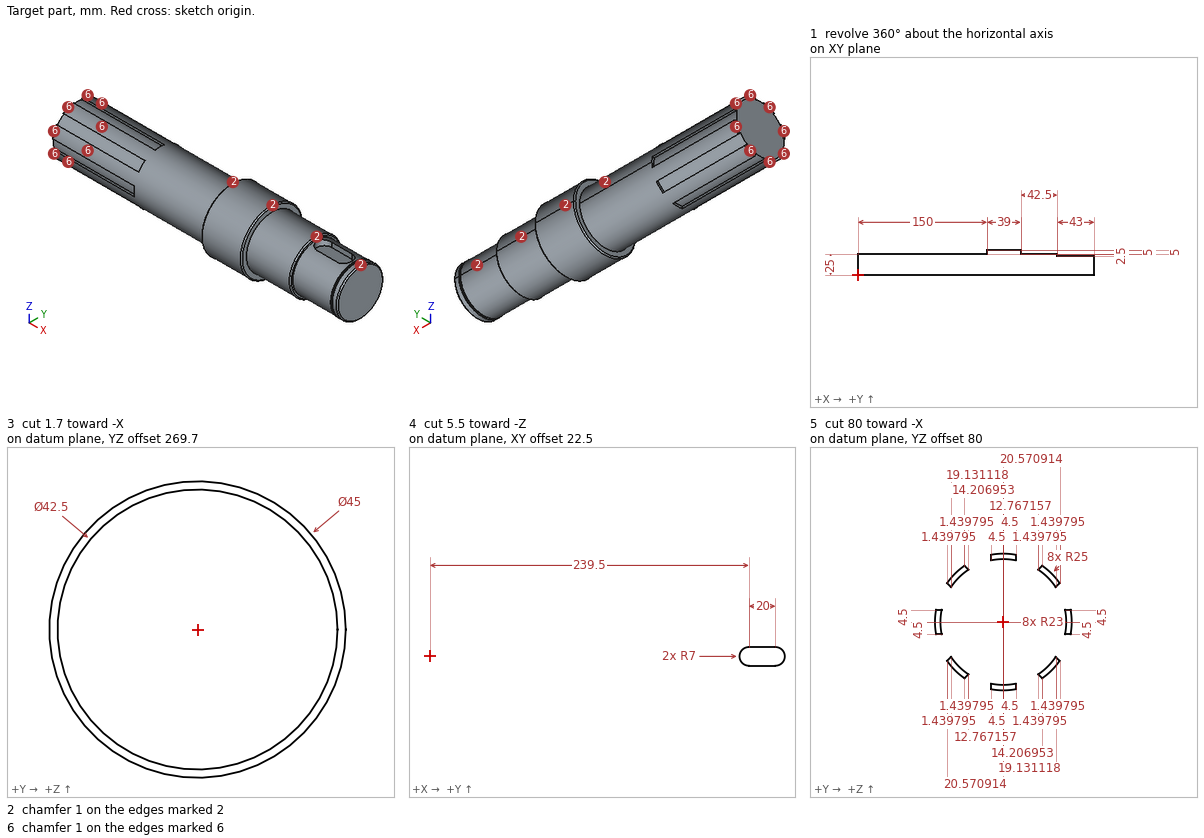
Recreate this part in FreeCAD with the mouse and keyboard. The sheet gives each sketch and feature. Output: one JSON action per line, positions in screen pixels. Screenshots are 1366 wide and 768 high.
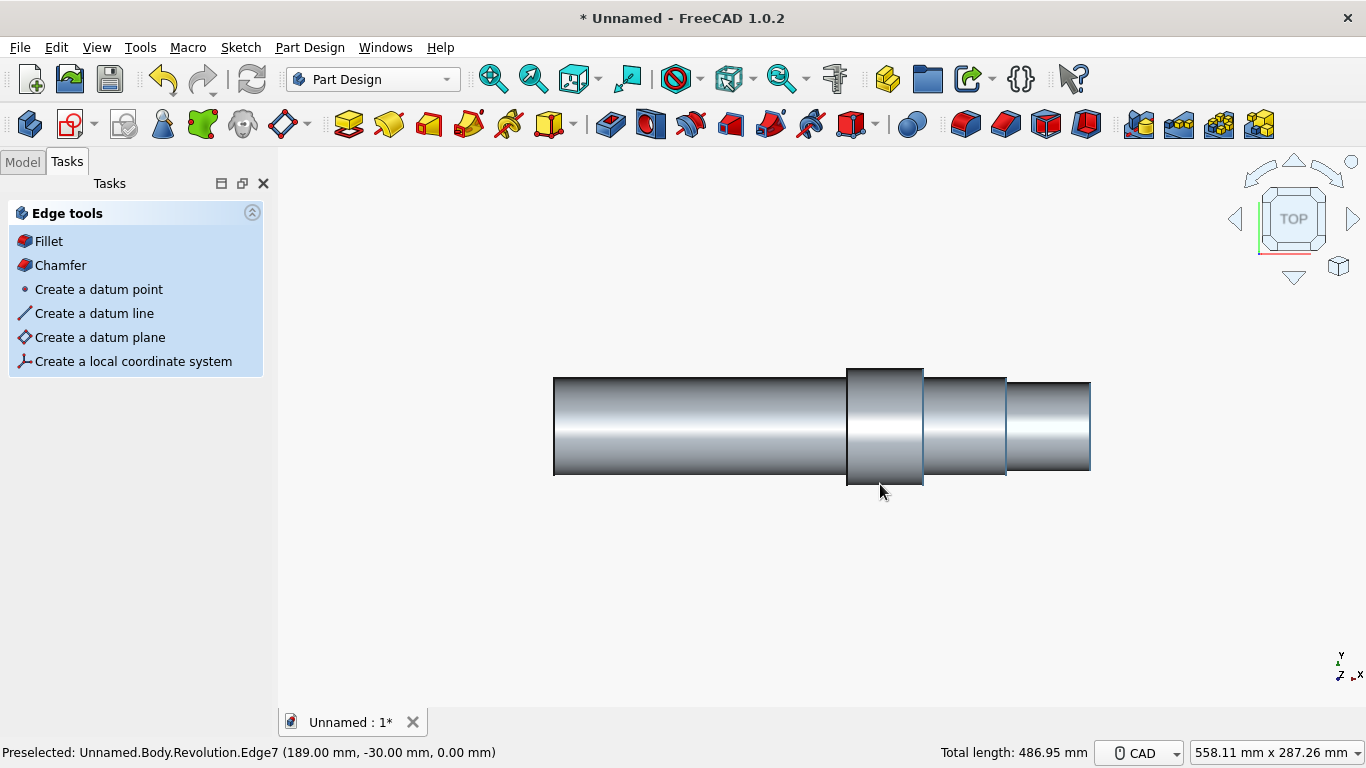
{"action": "left_click", "coordinate": [847, 473], "text": "ctrl"}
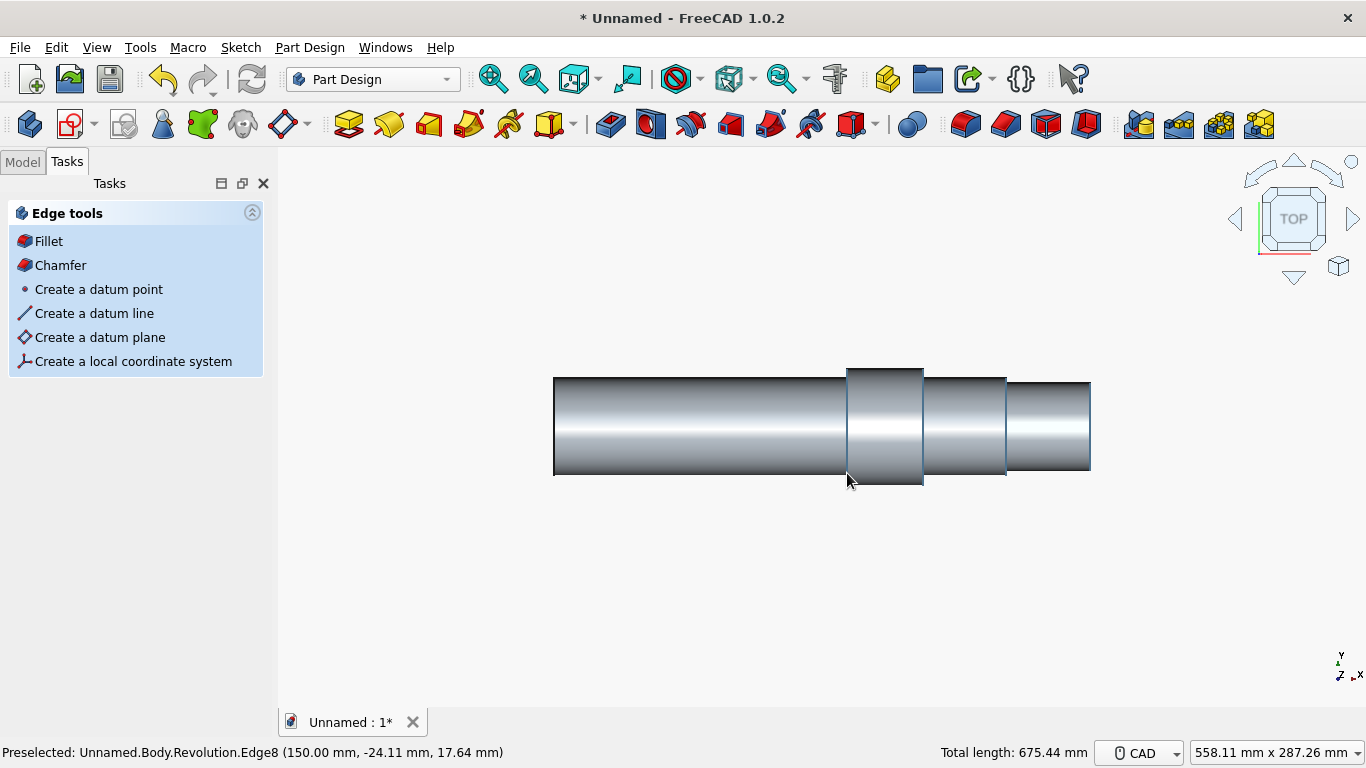
{"action": "left_click", "coordinate": [1006, 124]}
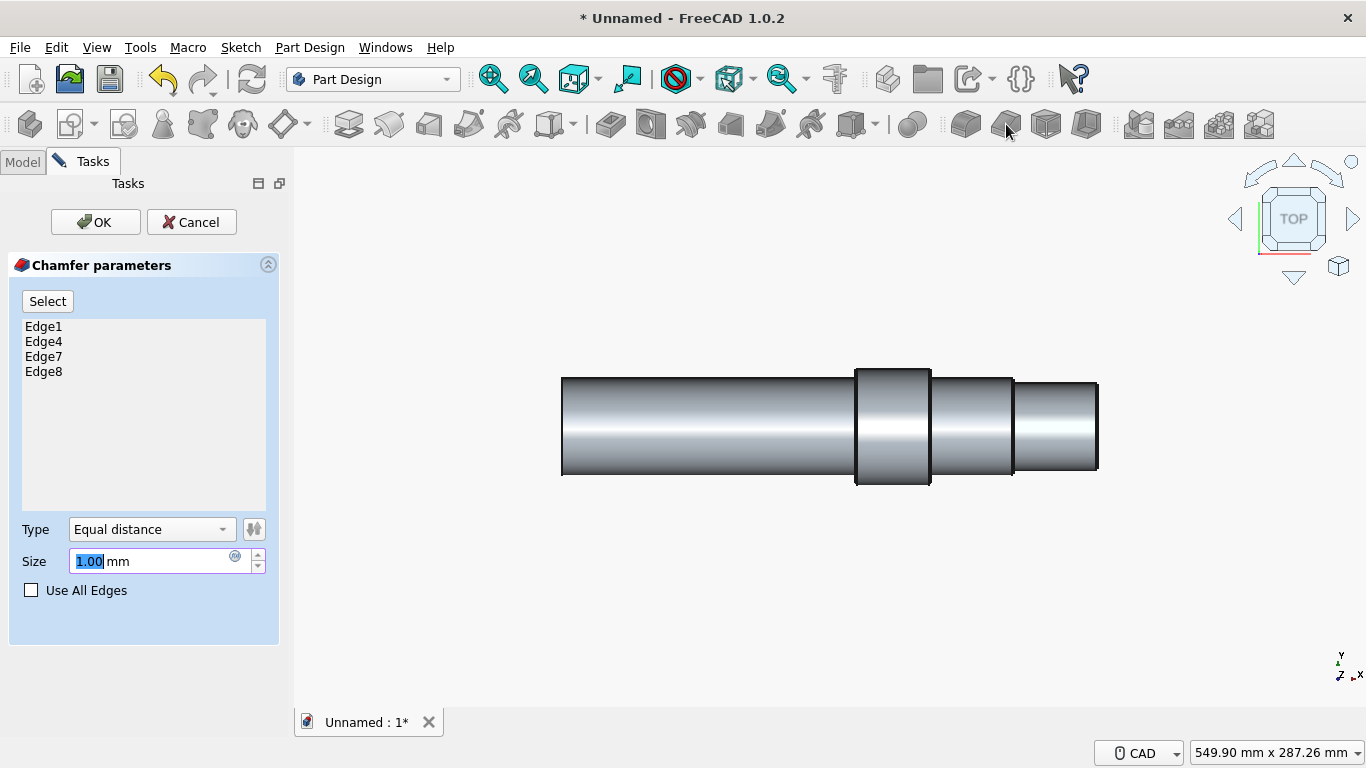
{"action": "type", "text": "1"}
{"action": "key", "text": "Tab"}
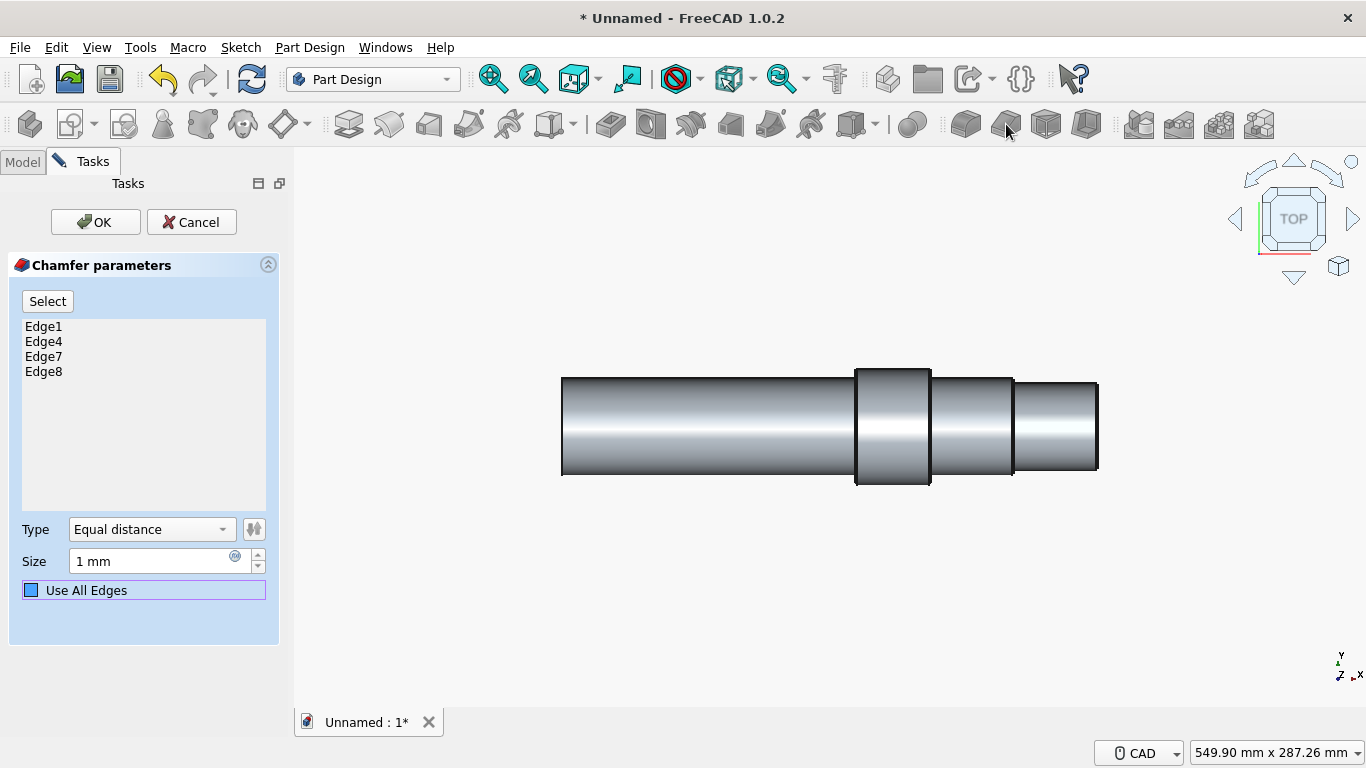
{"action": "left_click", "coordinate": [96, 222]}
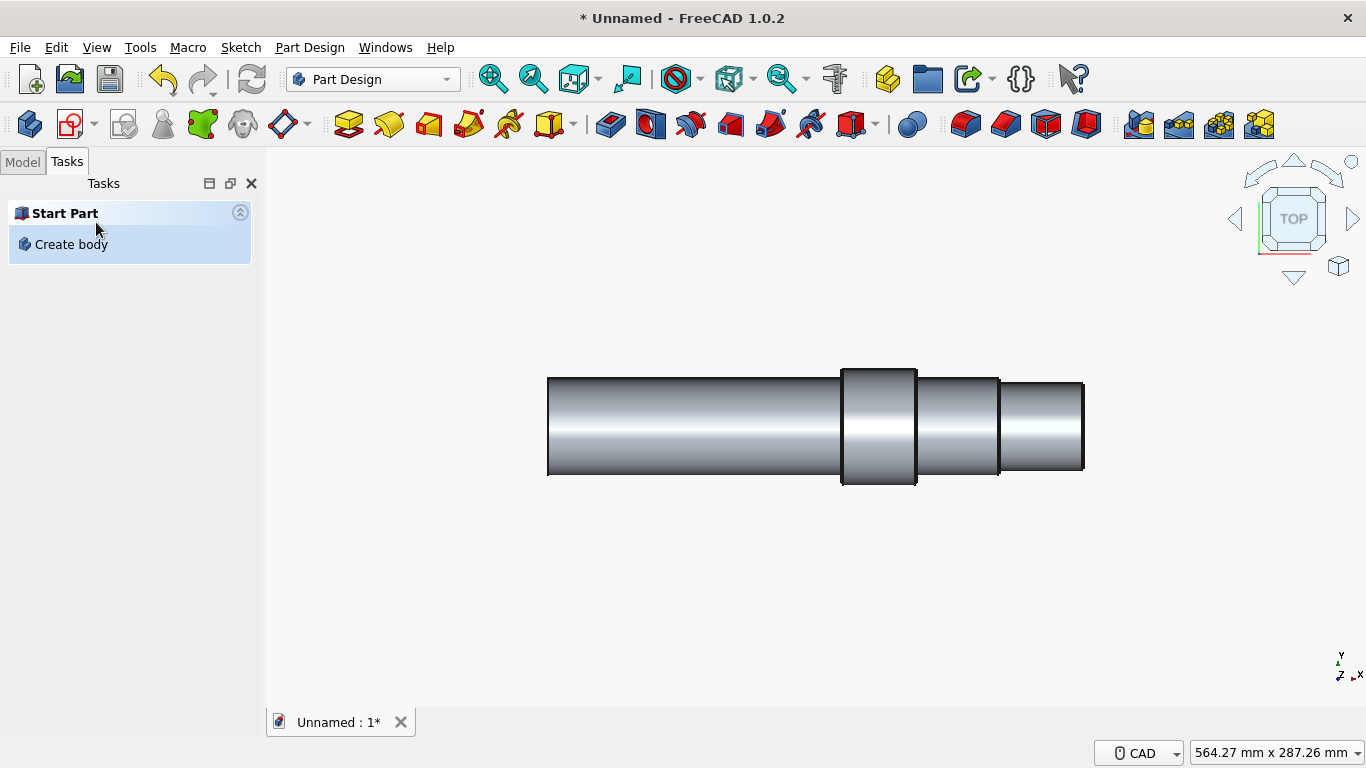
{"action": "left_click", "coordinate": [23, 161]}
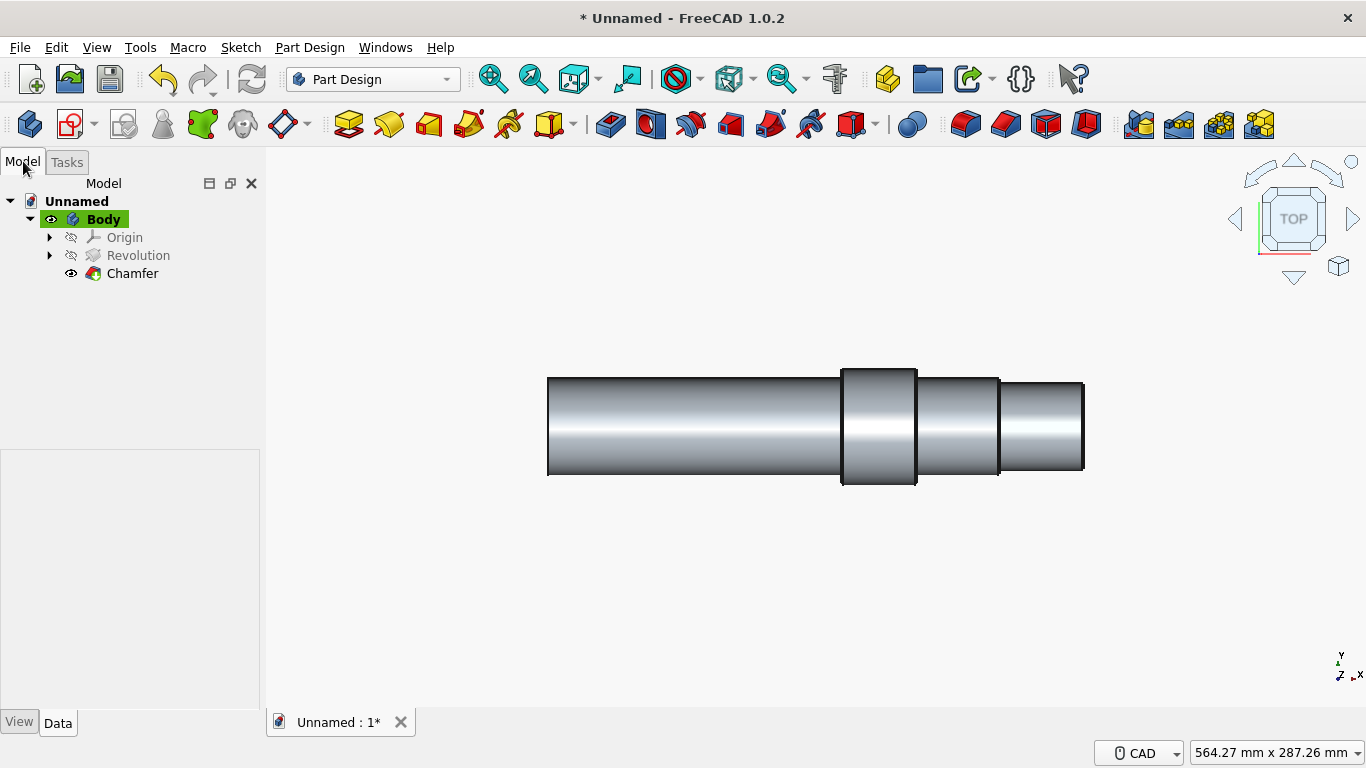
{"action": "left_click", "coordinate": [50, 237]}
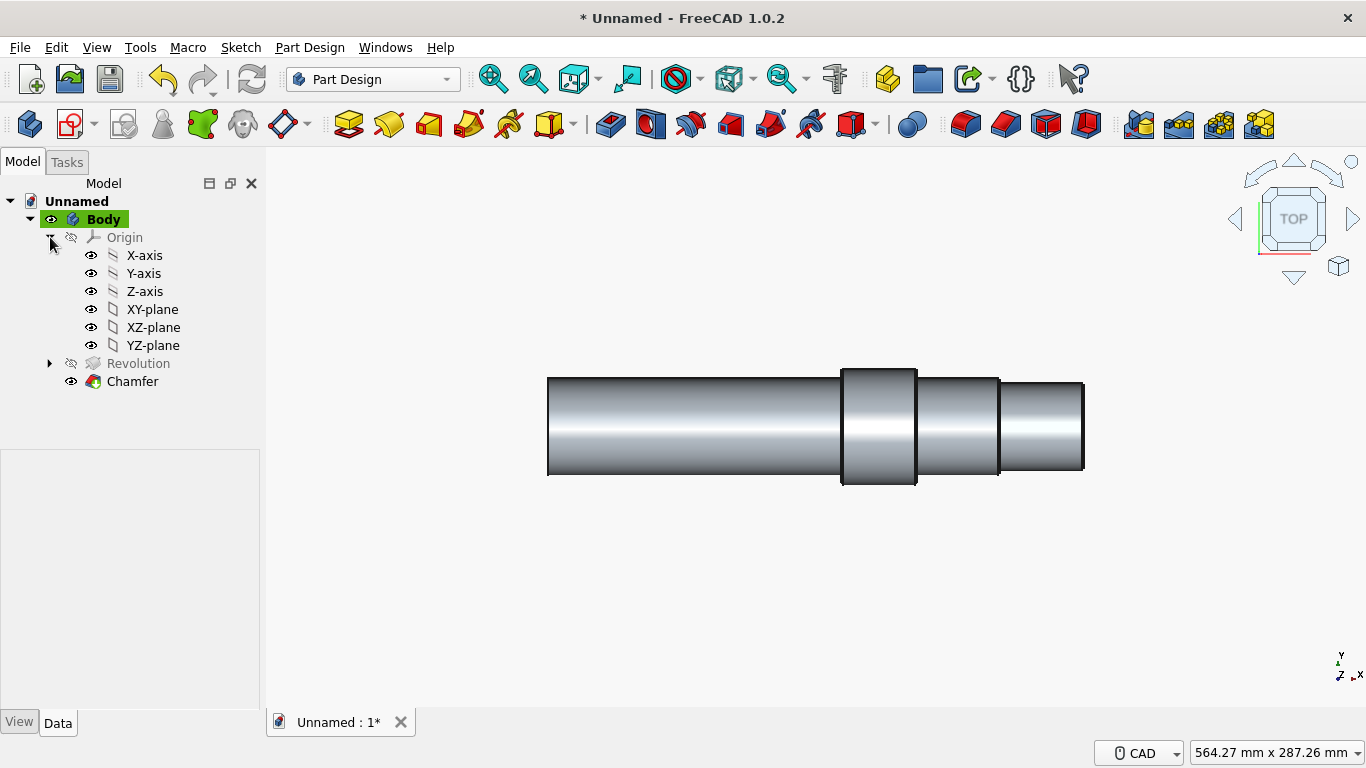
{"action": "left_click", "coordinate": [136, 345]}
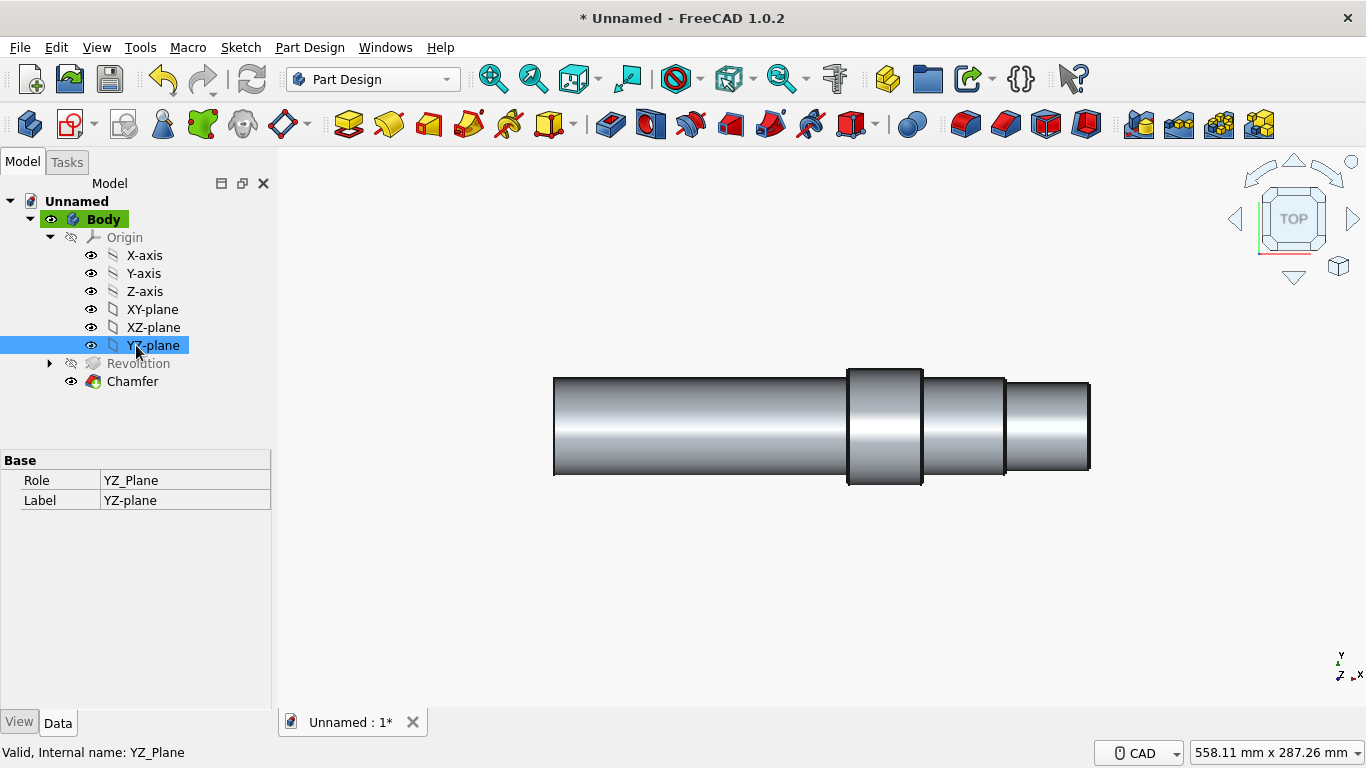
{"action": "left_click", "coordinate": [284, 124]}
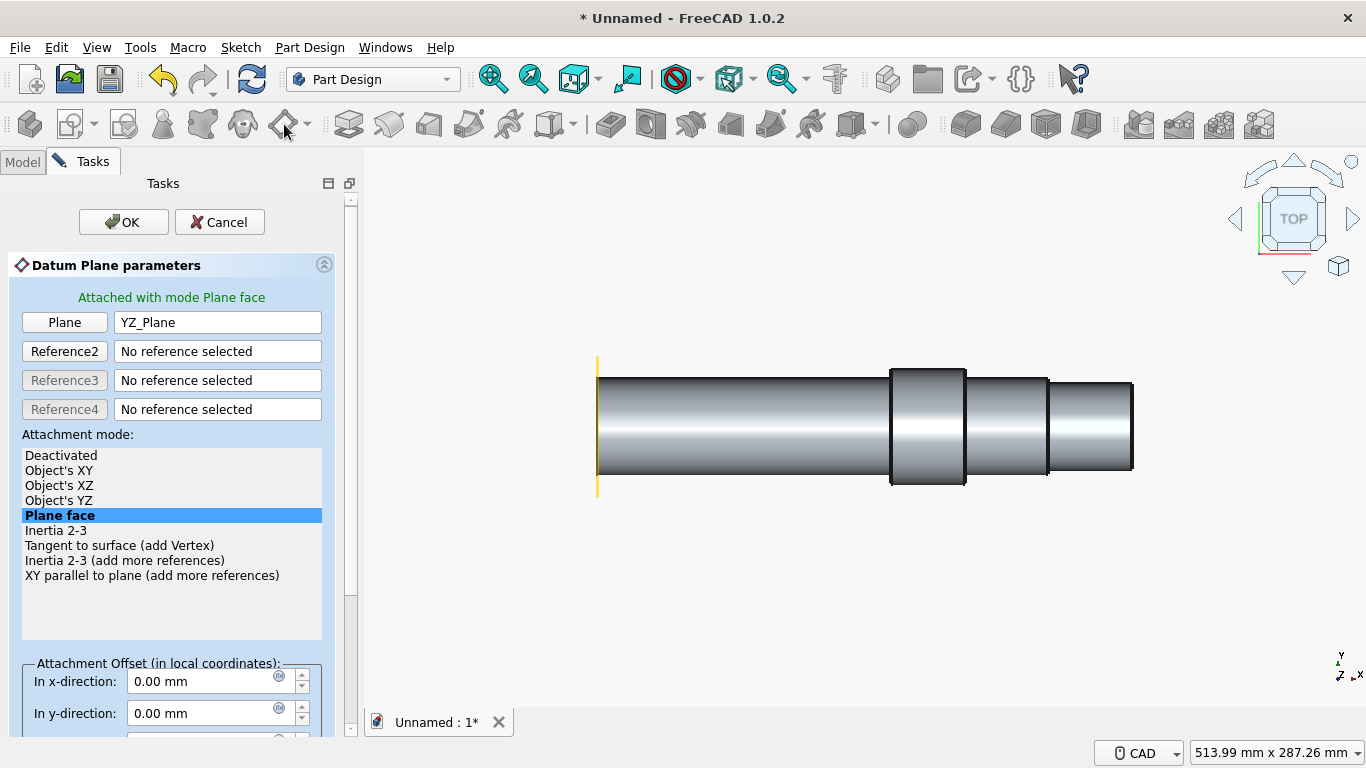
{"action": "scroll", "coordinate": [351, 464], "scroll_direction": "down", "scroll_amount": 2}